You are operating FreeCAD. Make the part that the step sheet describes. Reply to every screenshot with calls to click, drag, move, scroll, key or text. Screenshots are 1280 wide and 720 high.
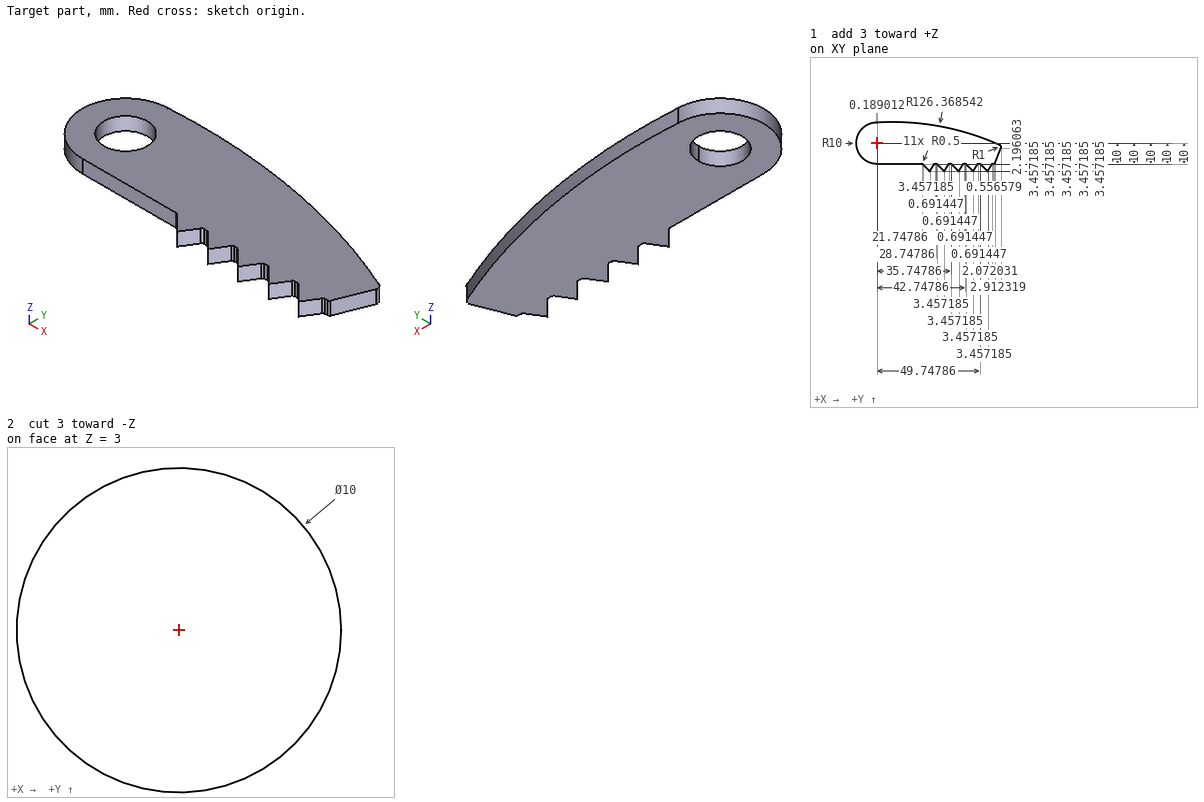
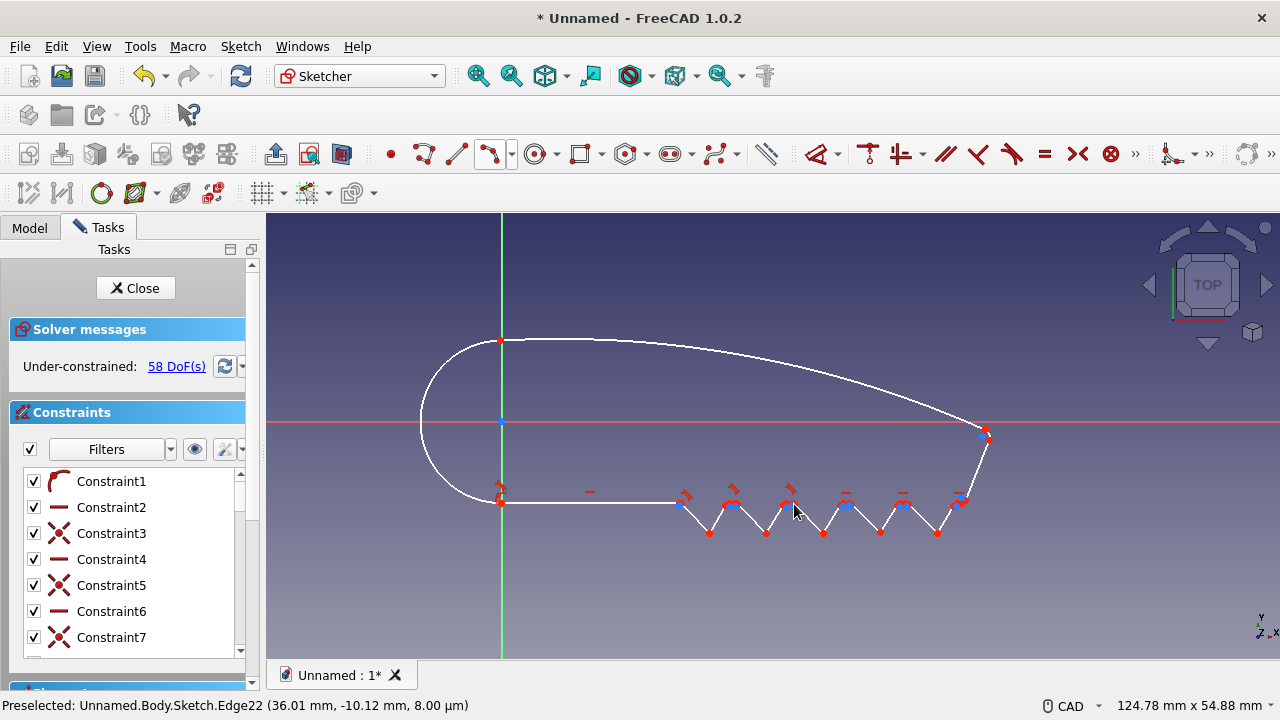
scroll(828, 525, up, 2)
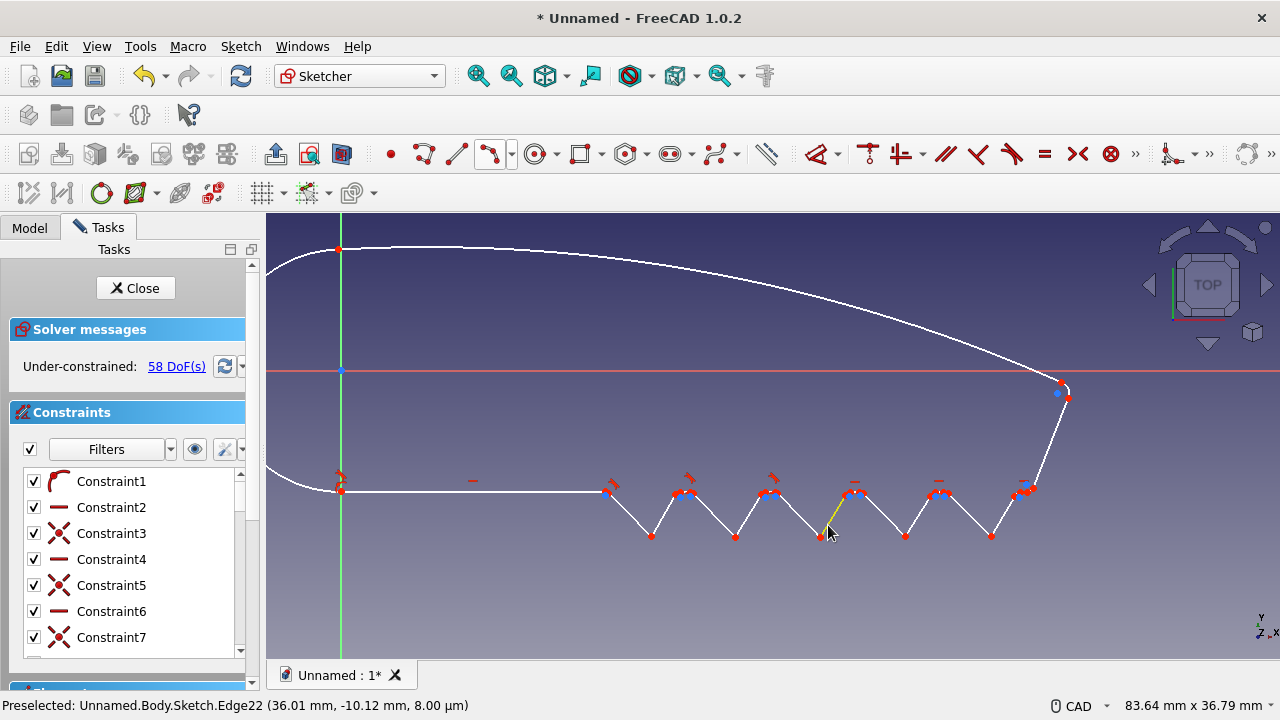
click(828, 525)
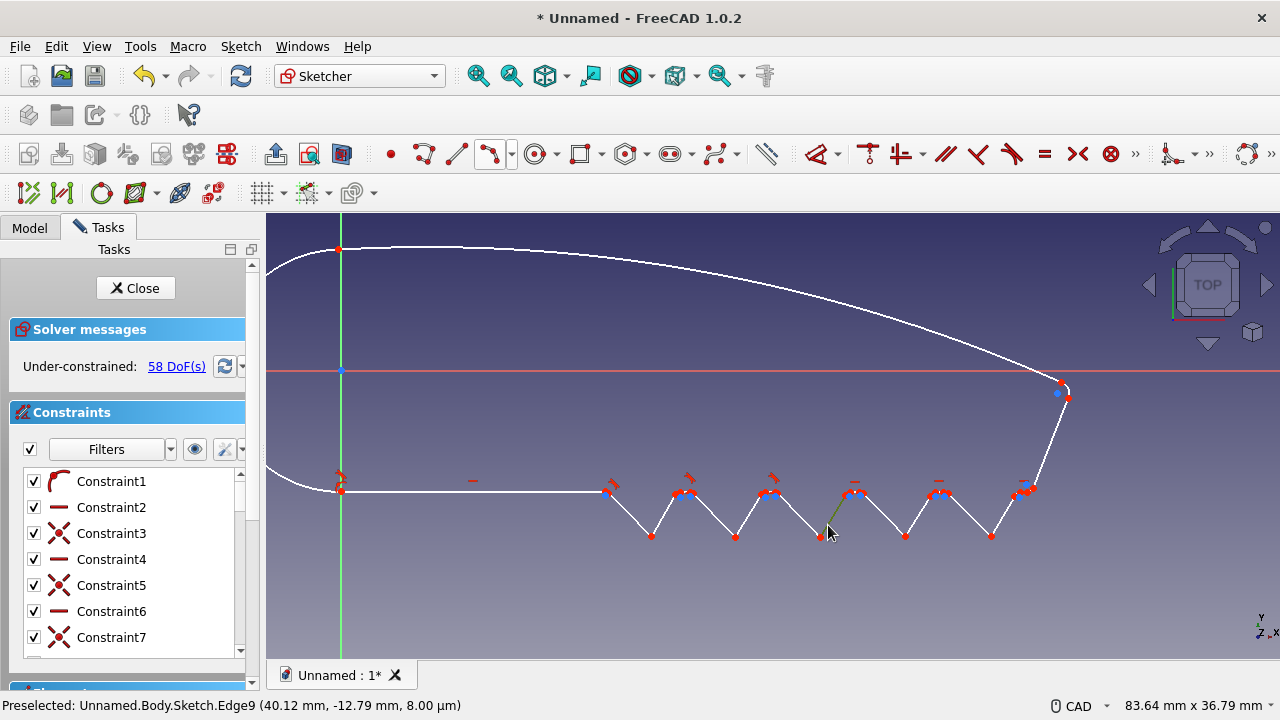
scroll(848, 493, up, 8)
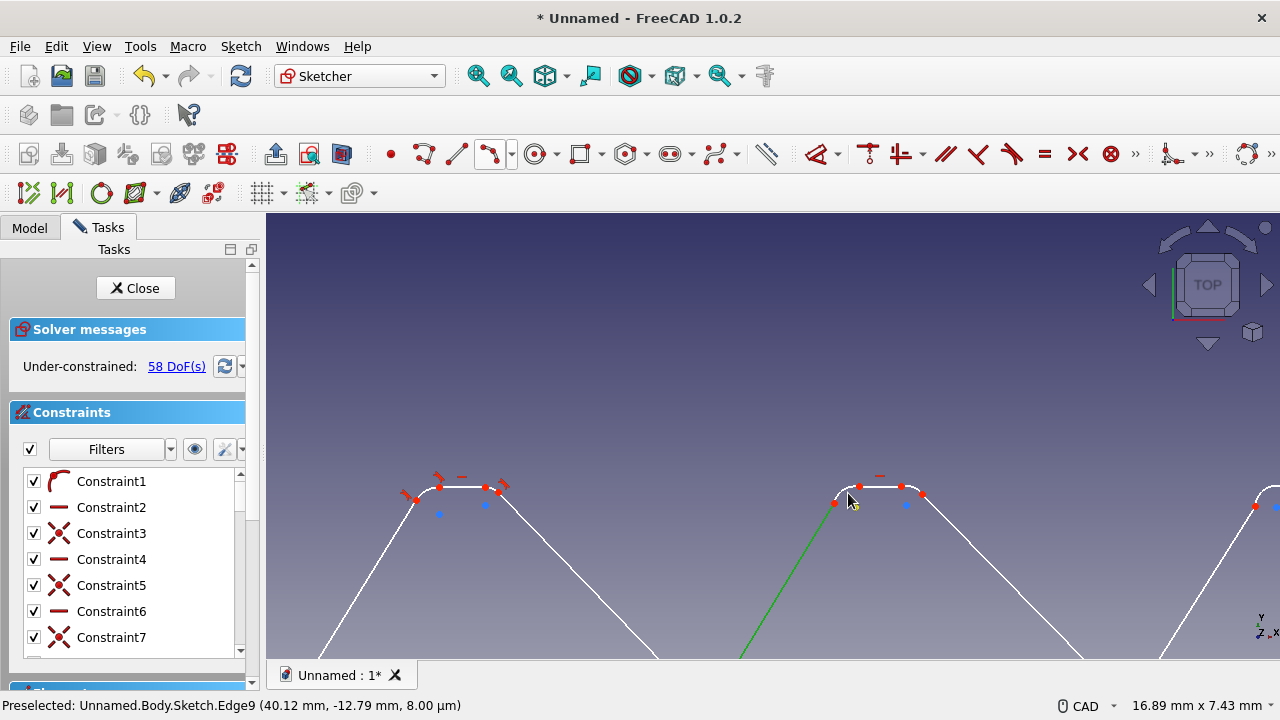
click(843, 490)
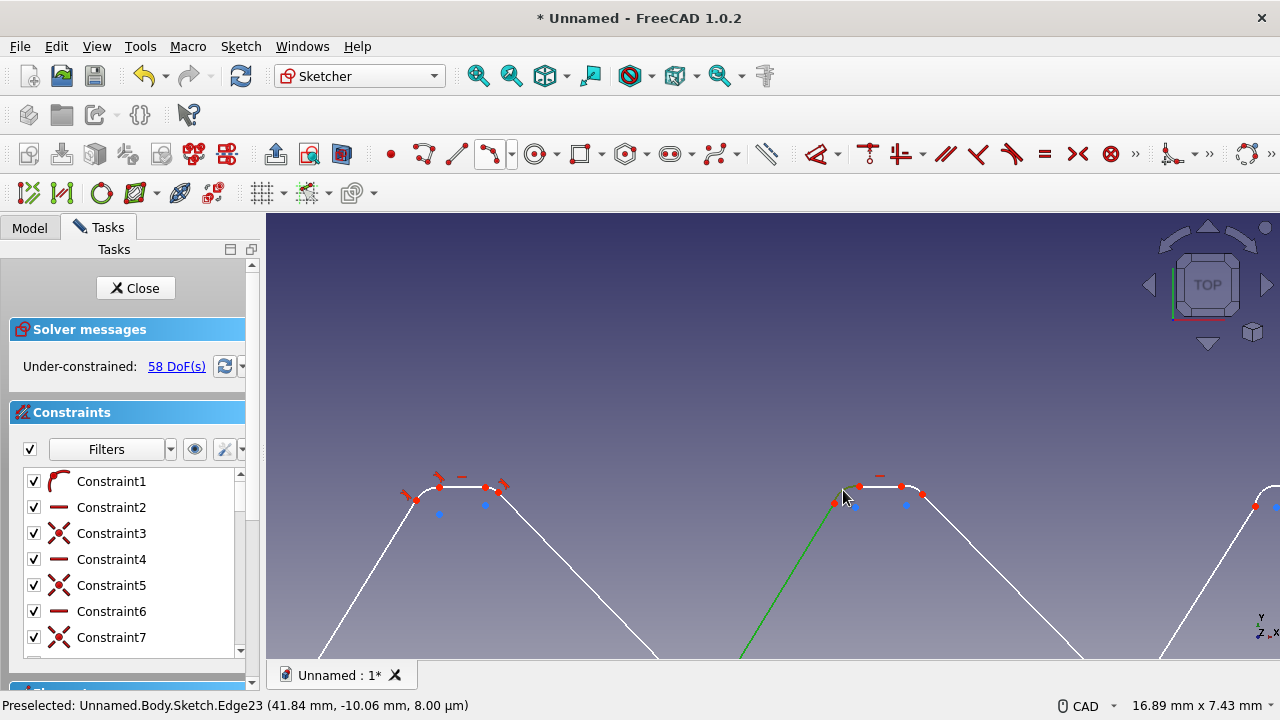
click(1012, 154)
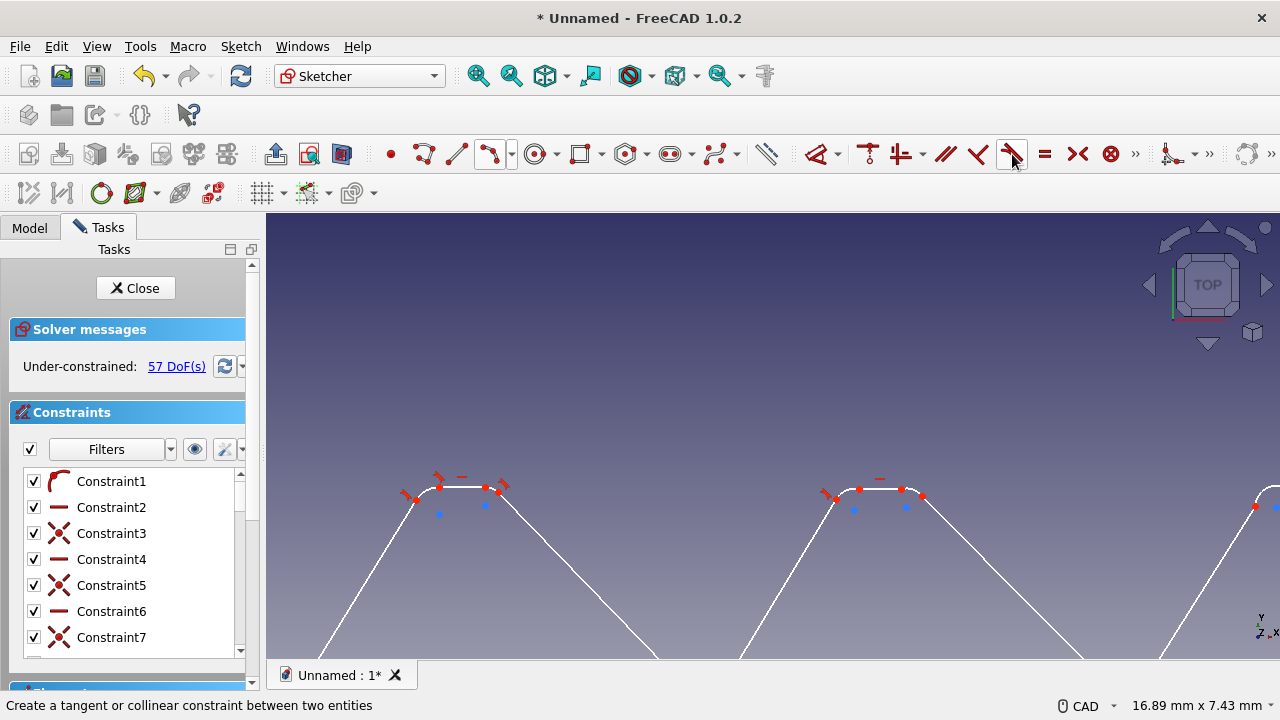
click(872, 489)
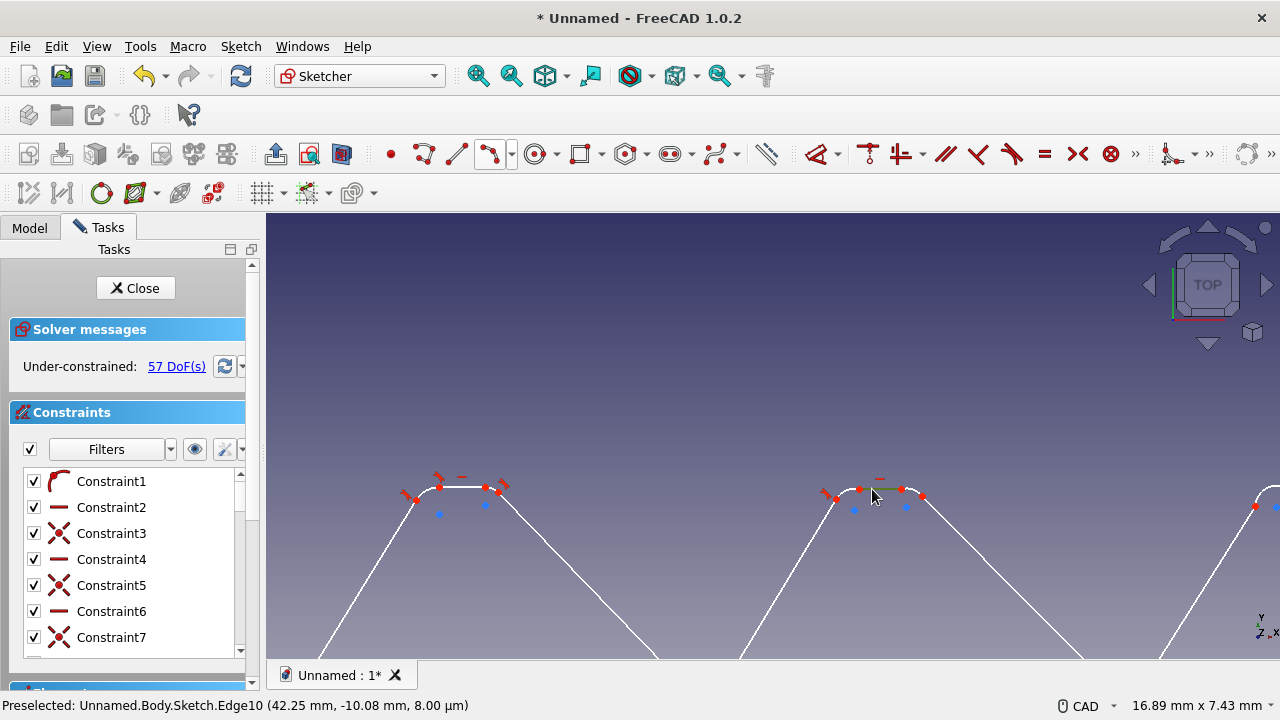
click(846, 491)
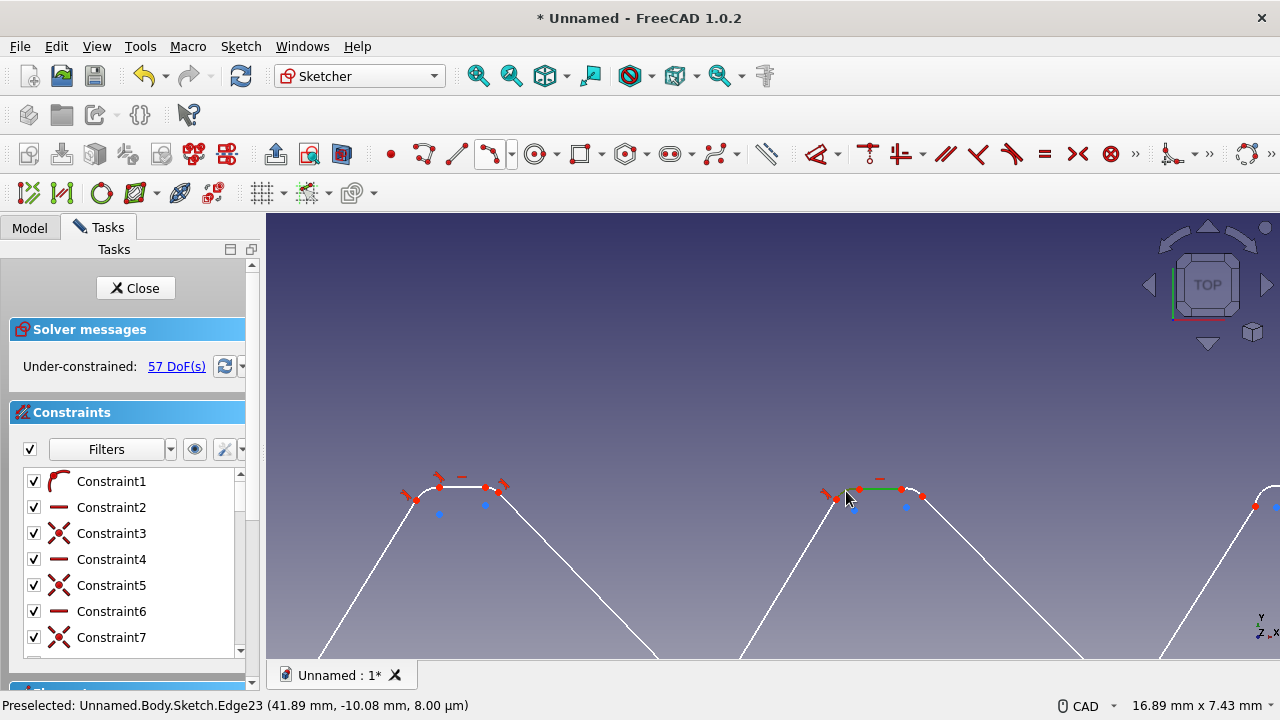
click(1012, 154)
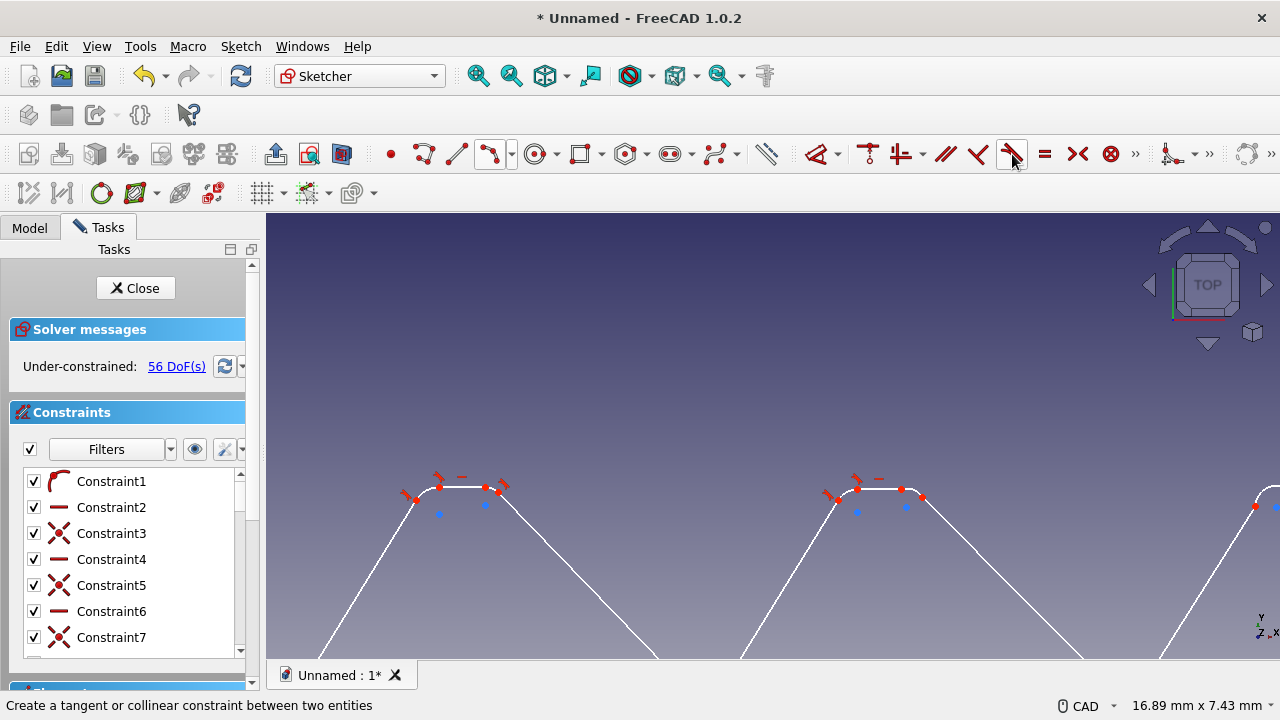
click(871, 489)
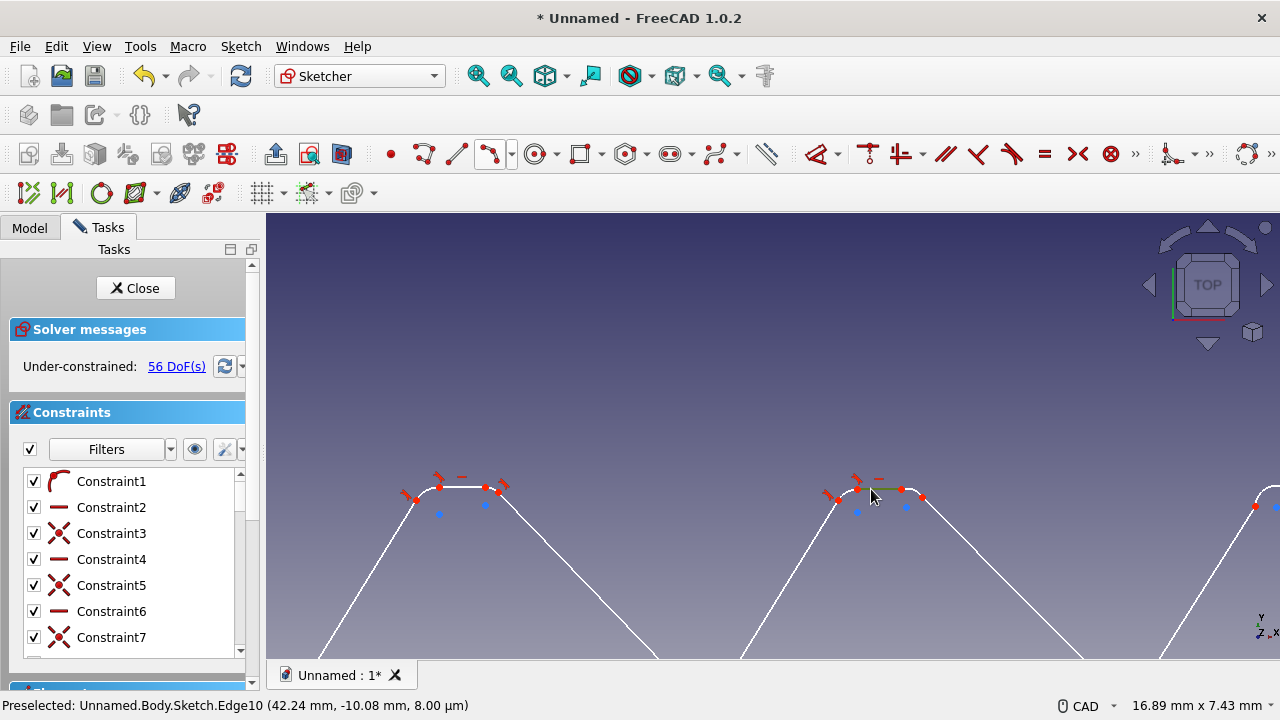
click(913, 490)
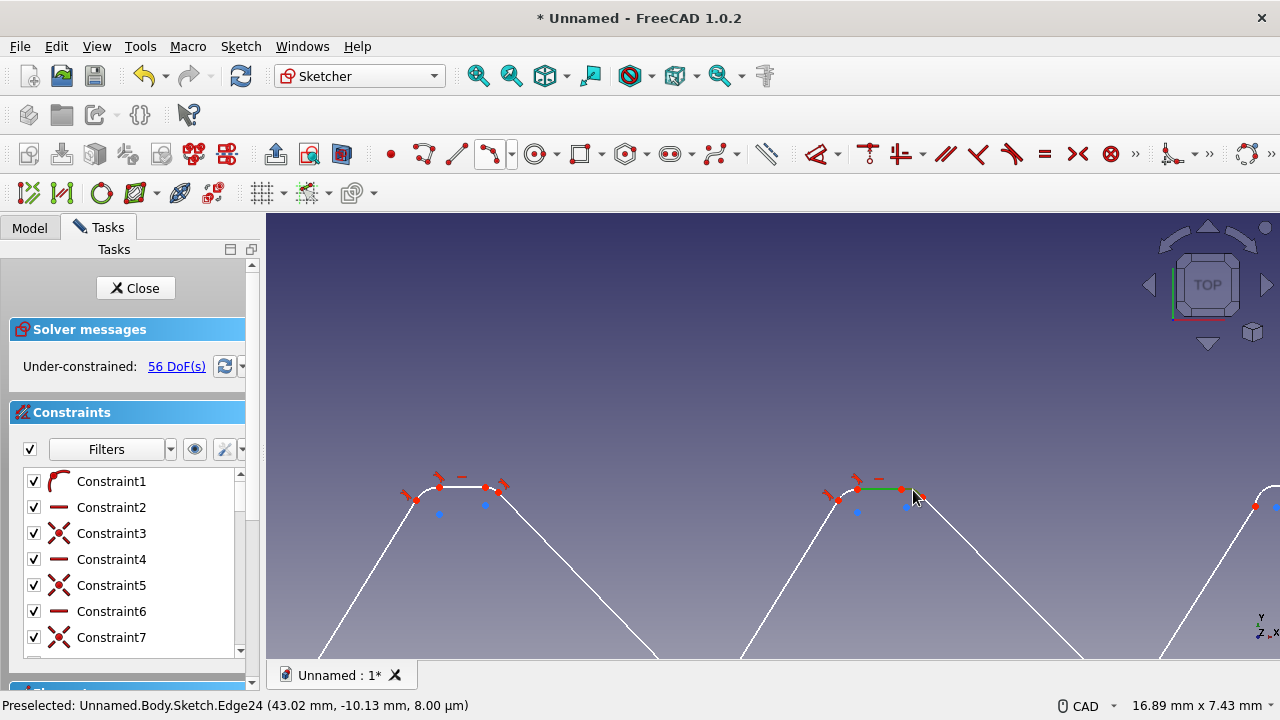
click(1012, 154)